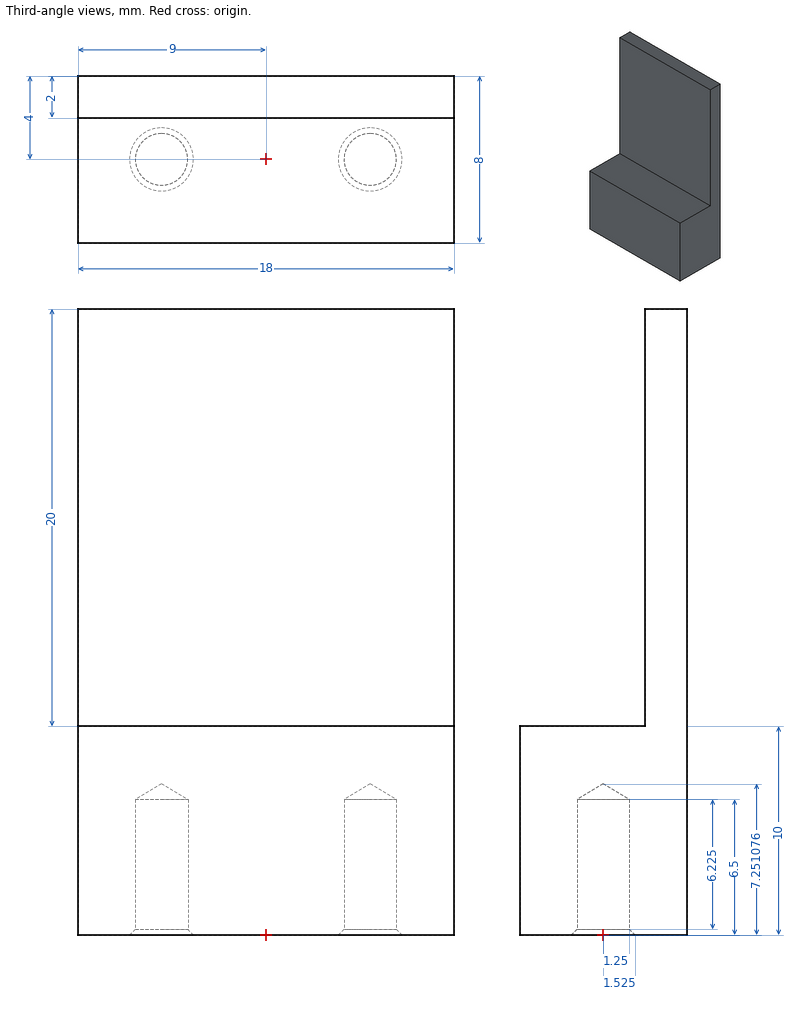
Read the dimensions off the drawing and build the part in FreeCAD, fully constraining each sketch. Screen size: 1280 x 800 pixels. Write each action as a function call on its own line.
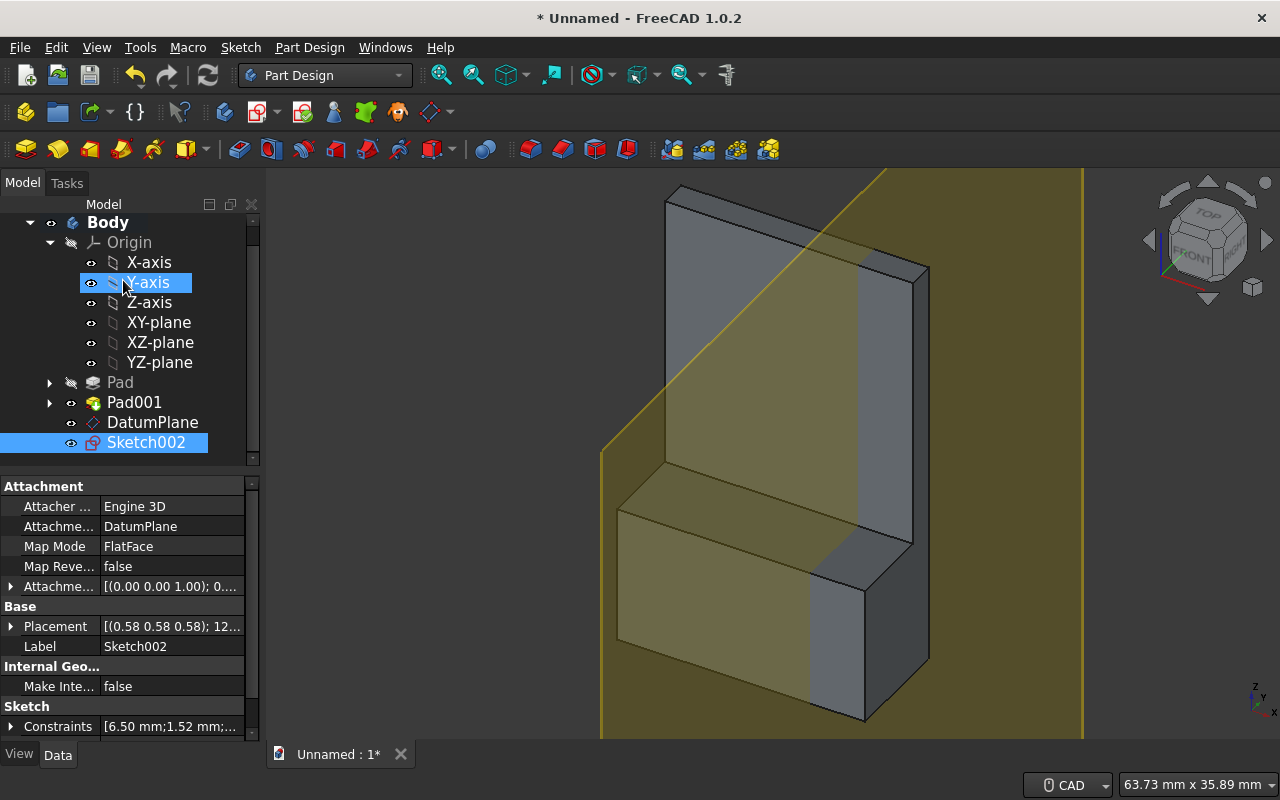
click(304, 150)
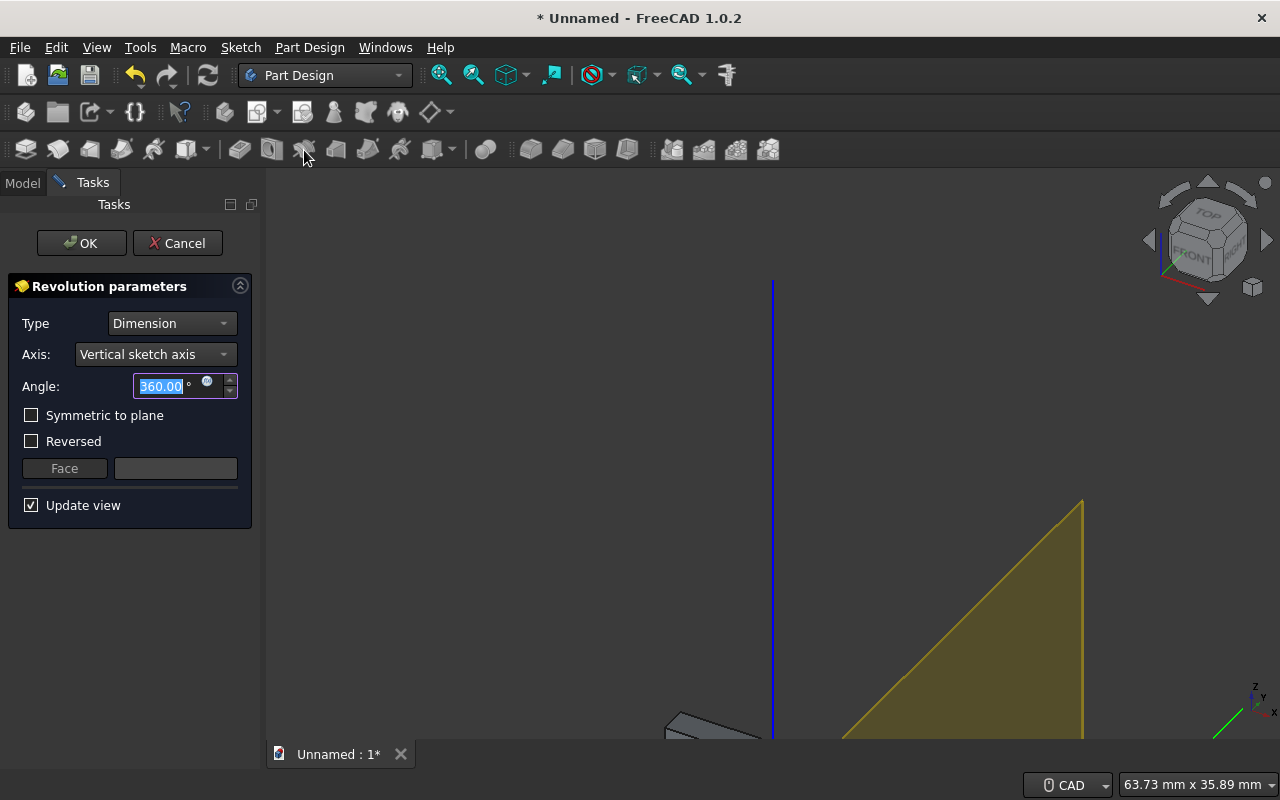
click(82, 243)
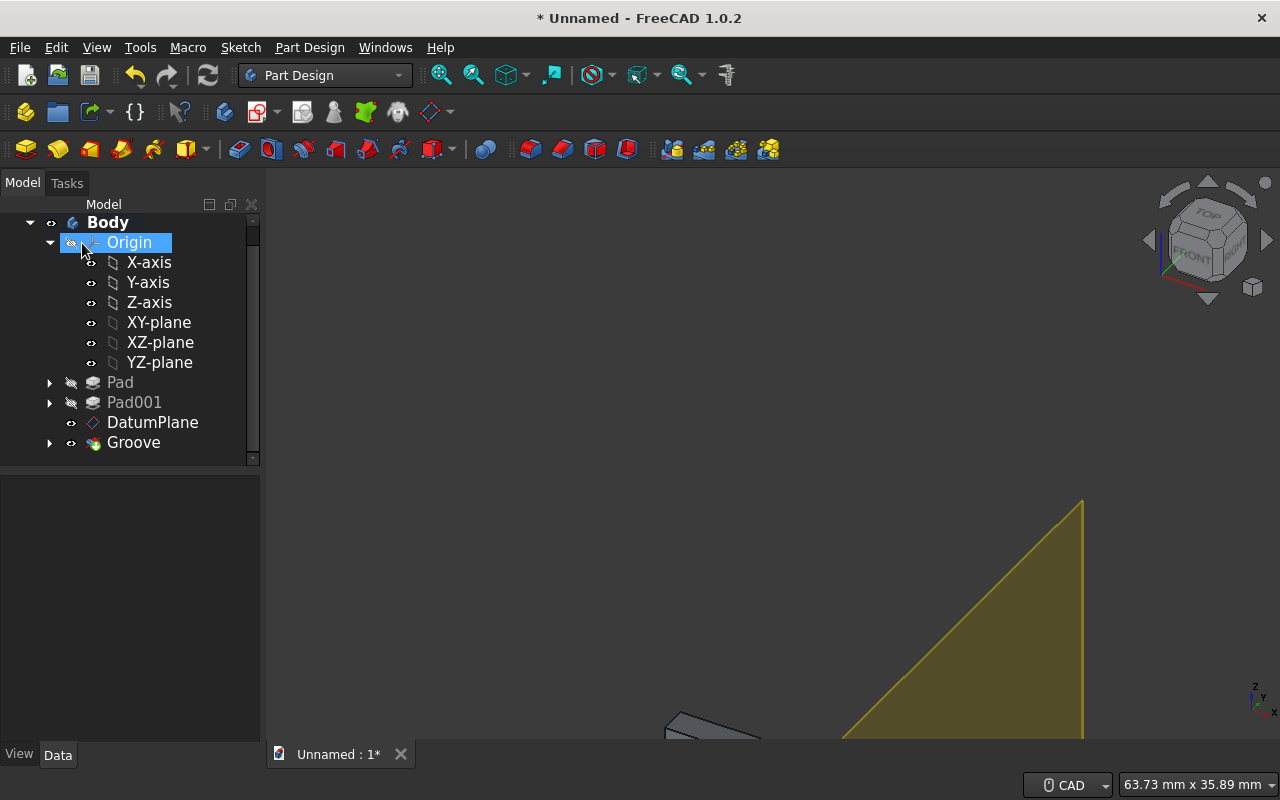
click(116, 423)
key(space)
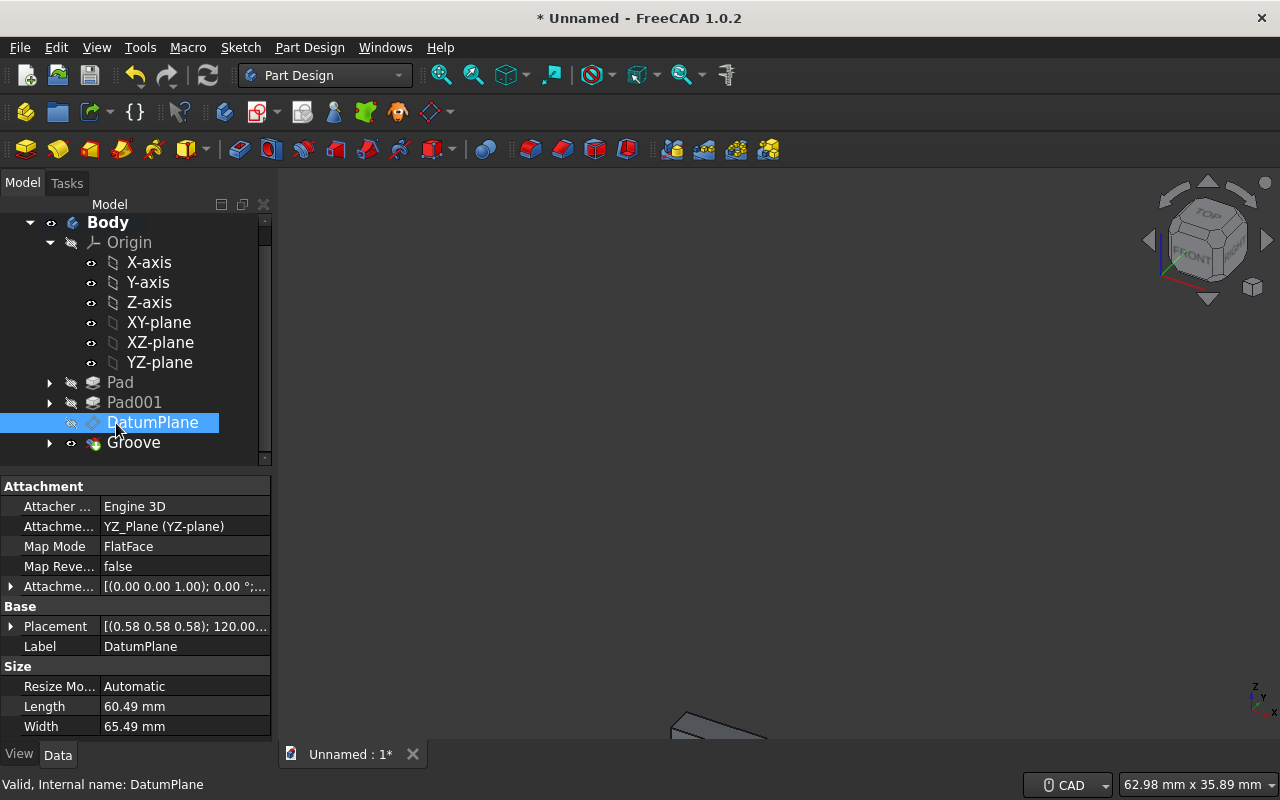
click(442, 76)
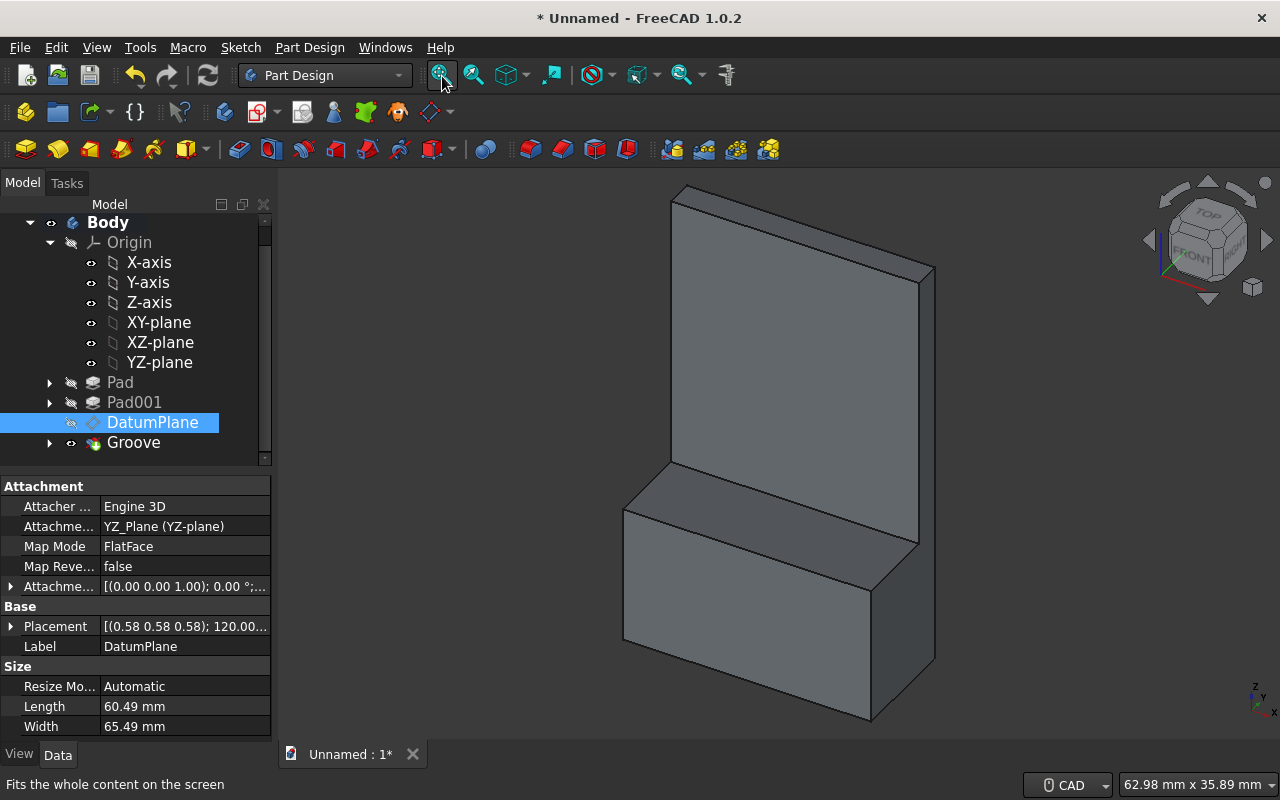
click(116, 443)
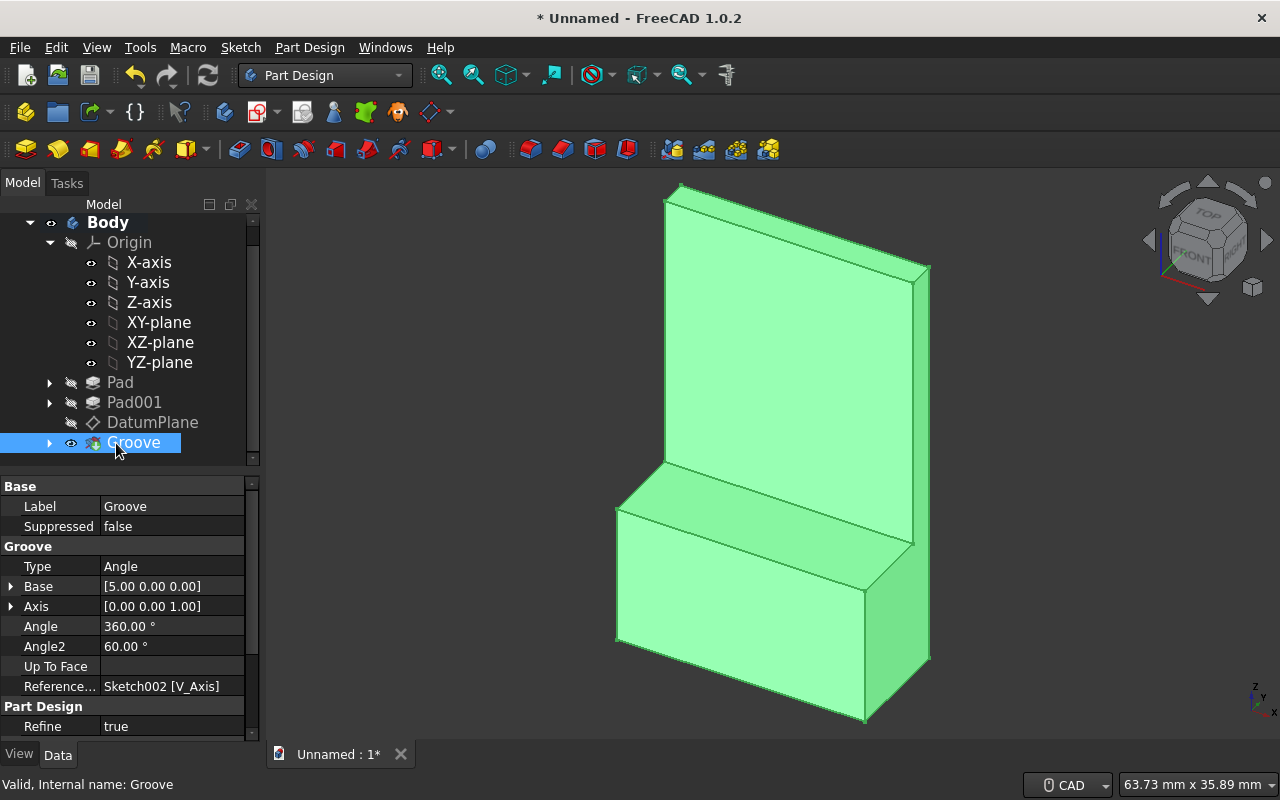
click(672, 150)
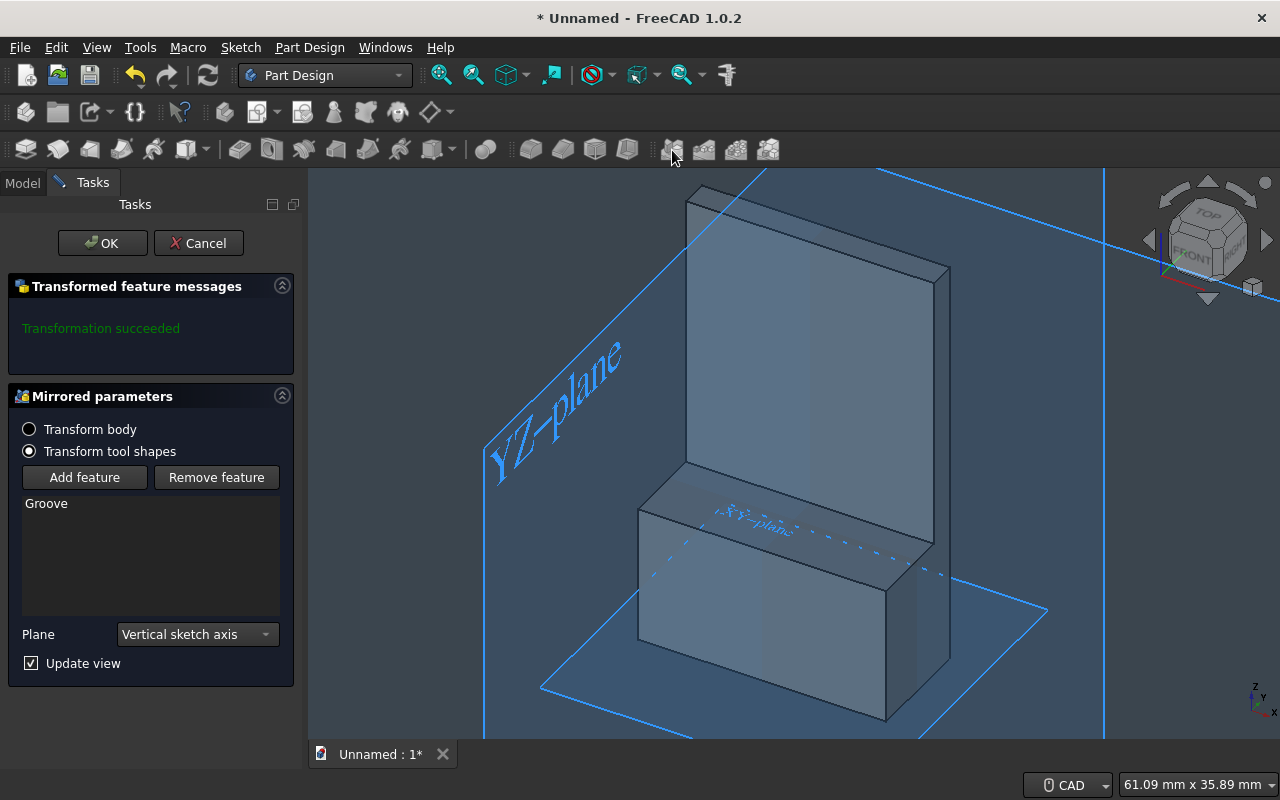
click(198, 634)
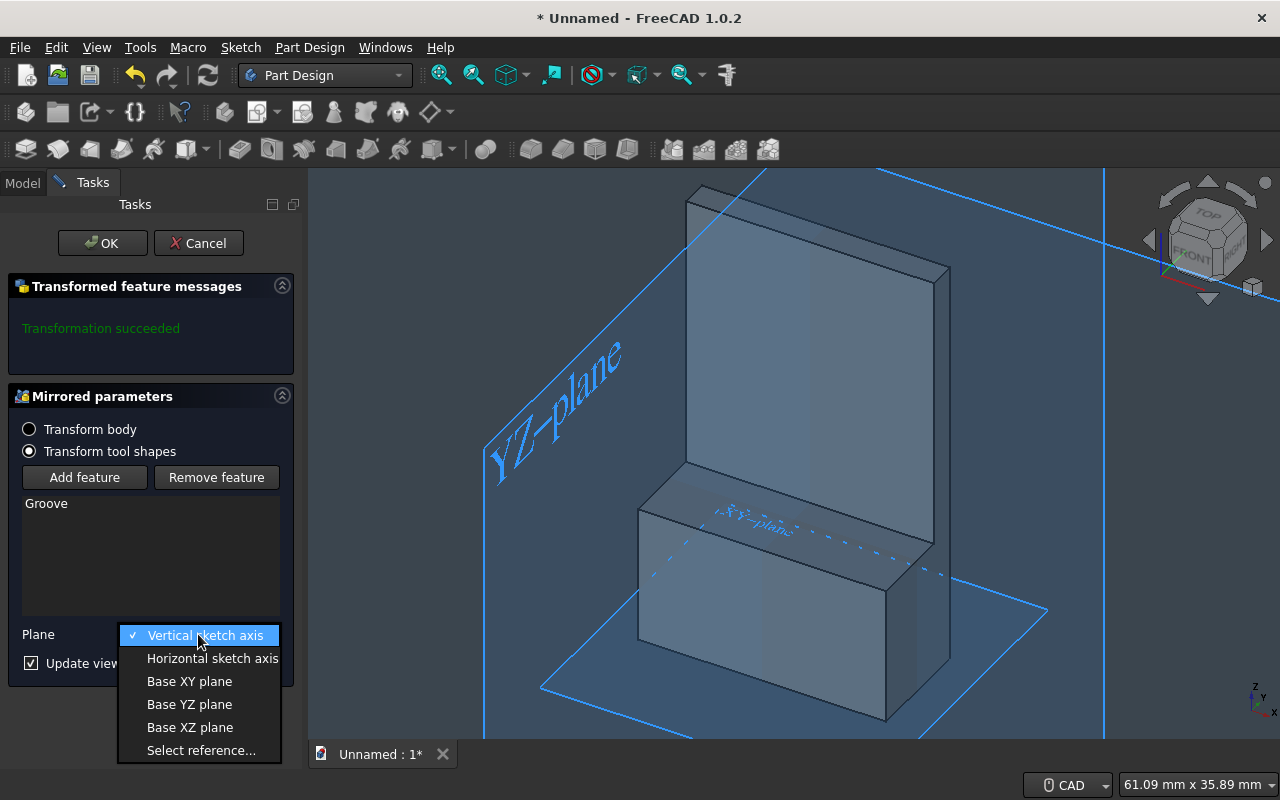
click(198, 704)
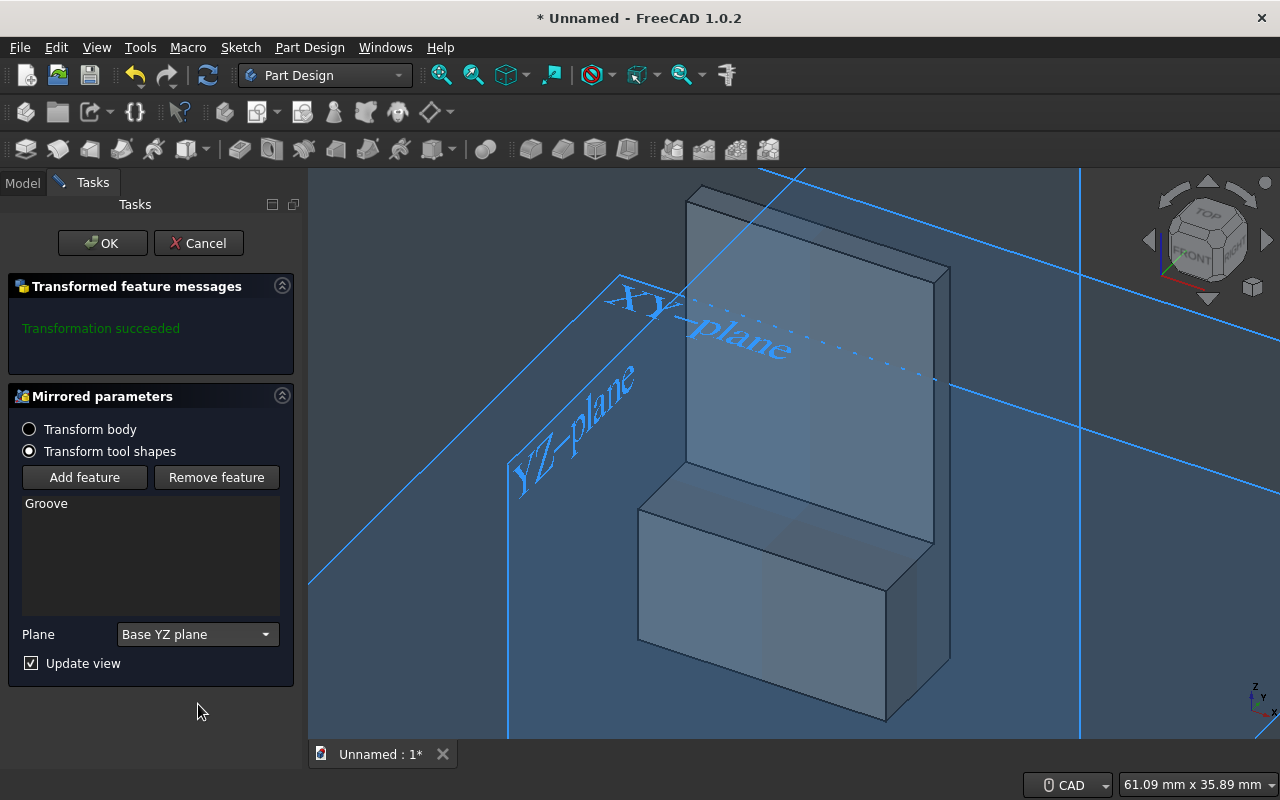
click(103, 243)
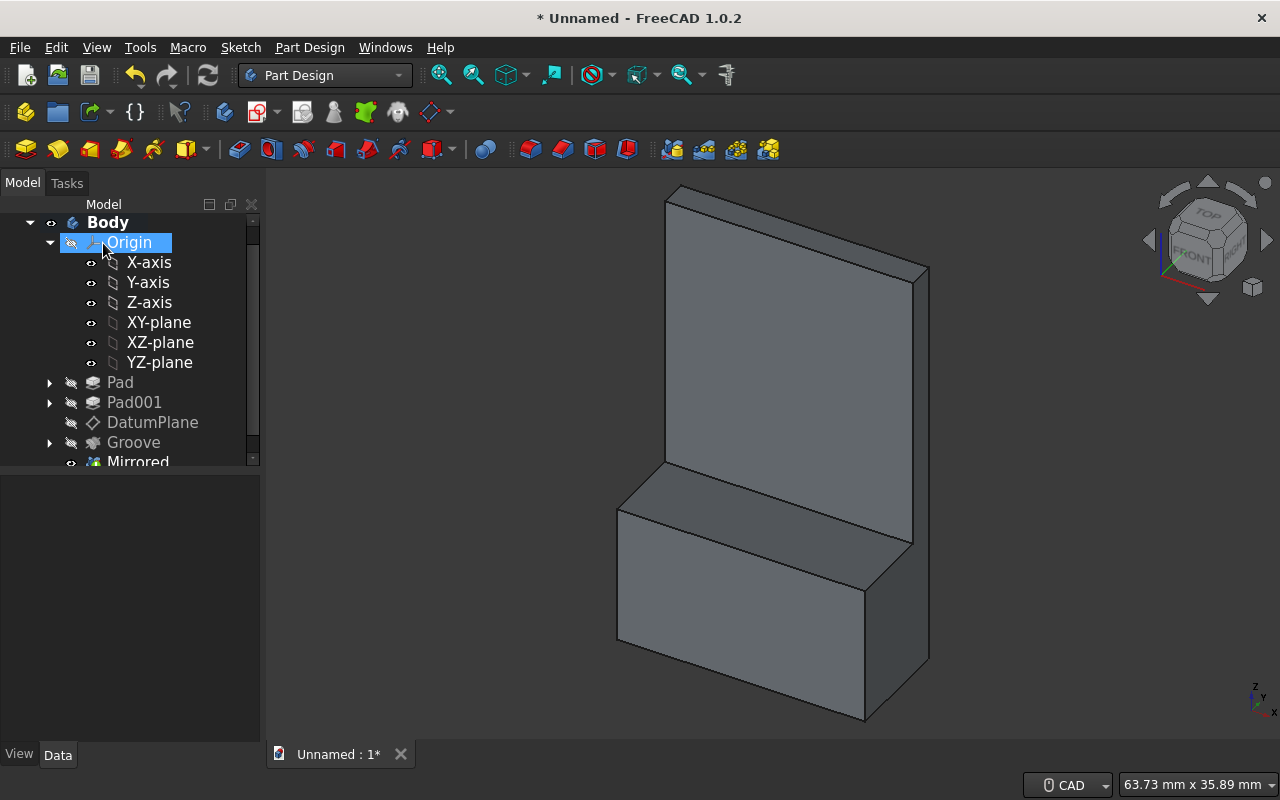
key(0)